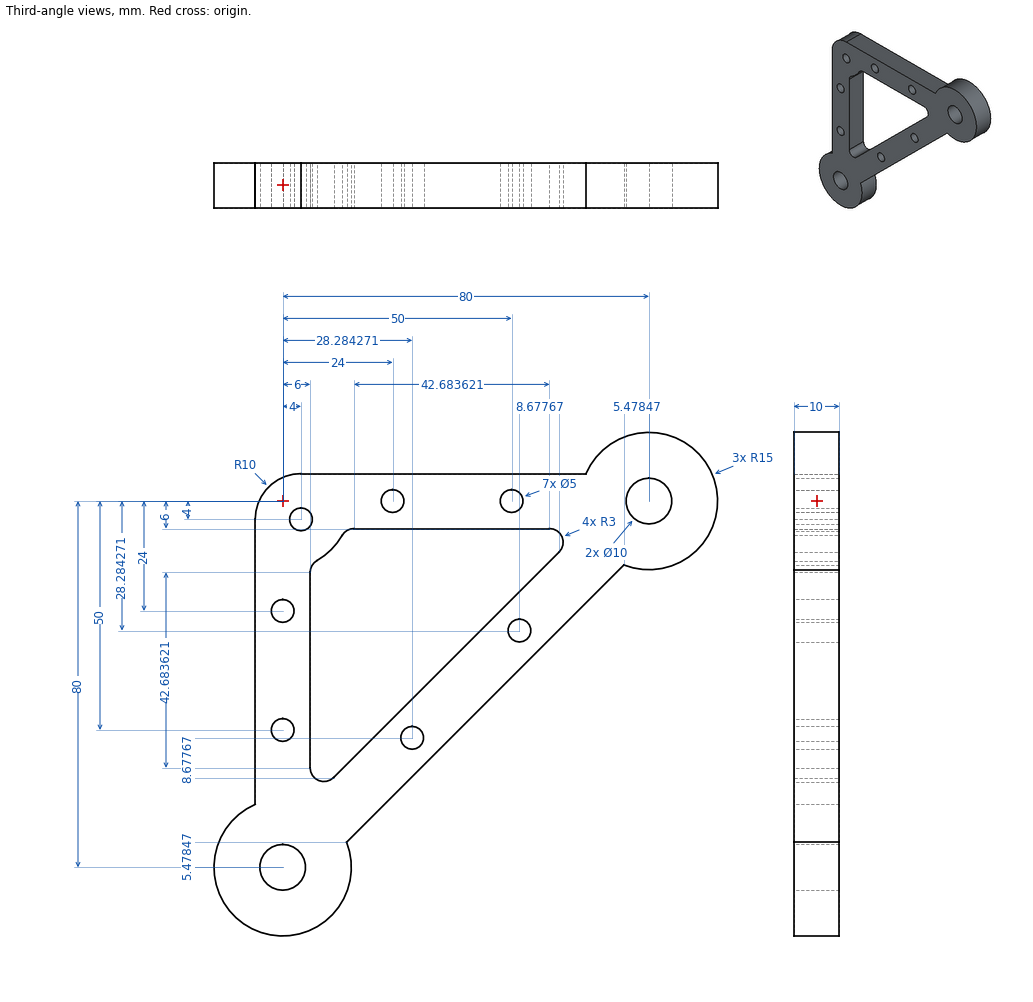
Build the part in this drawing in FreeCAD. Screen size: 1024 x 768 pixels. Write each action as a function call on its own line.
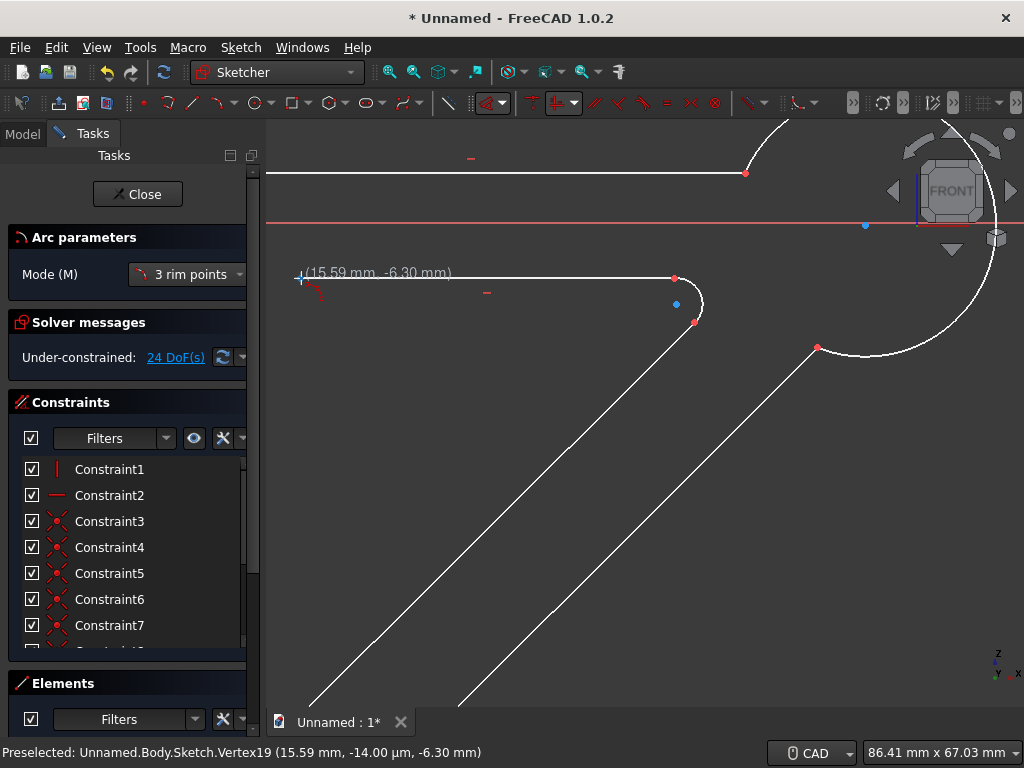
scroll(599, 254, down, 4)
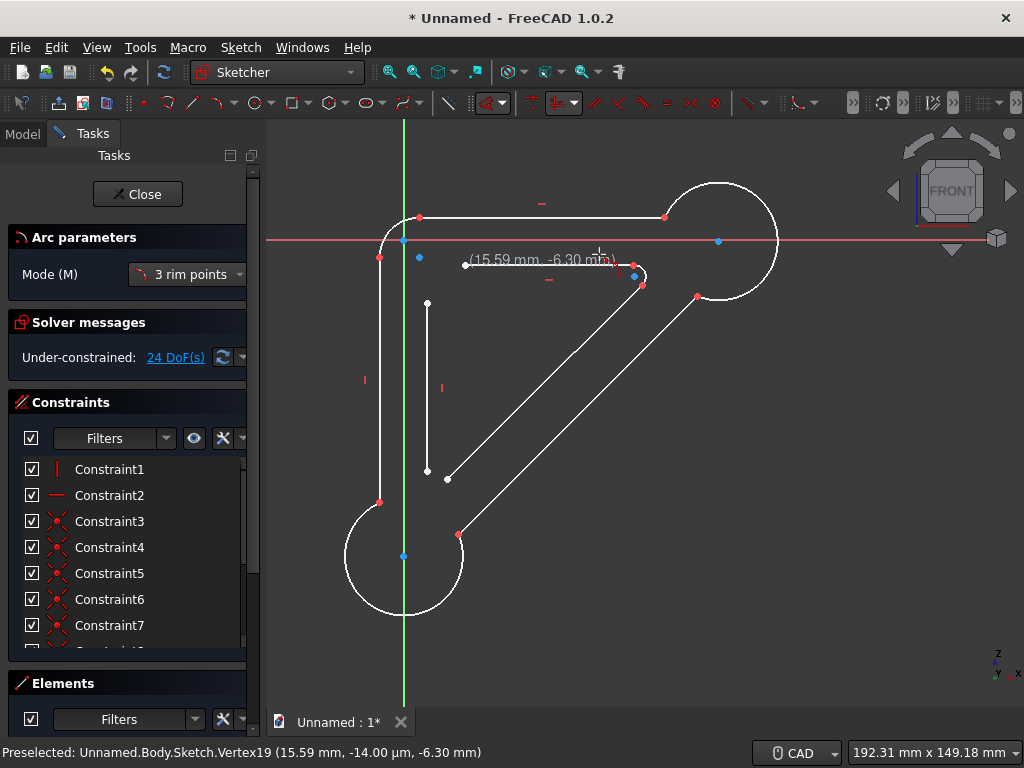
scroll(455, 270, up, 2)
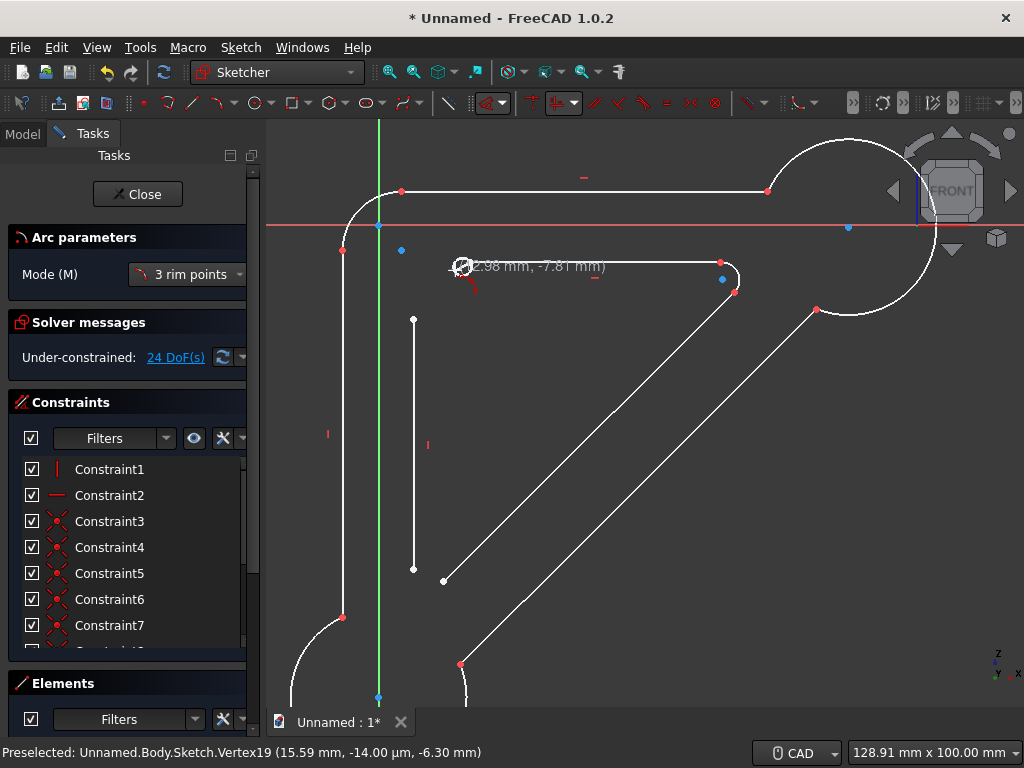
click(455, 270)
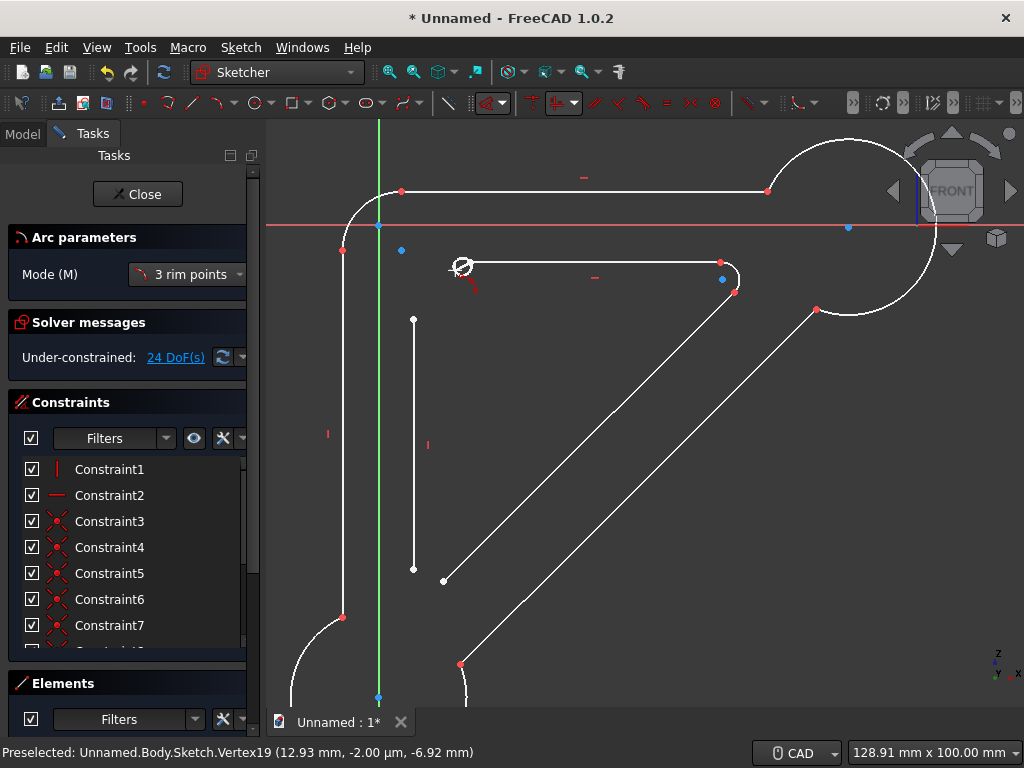
scroll(461, 263, up, 10)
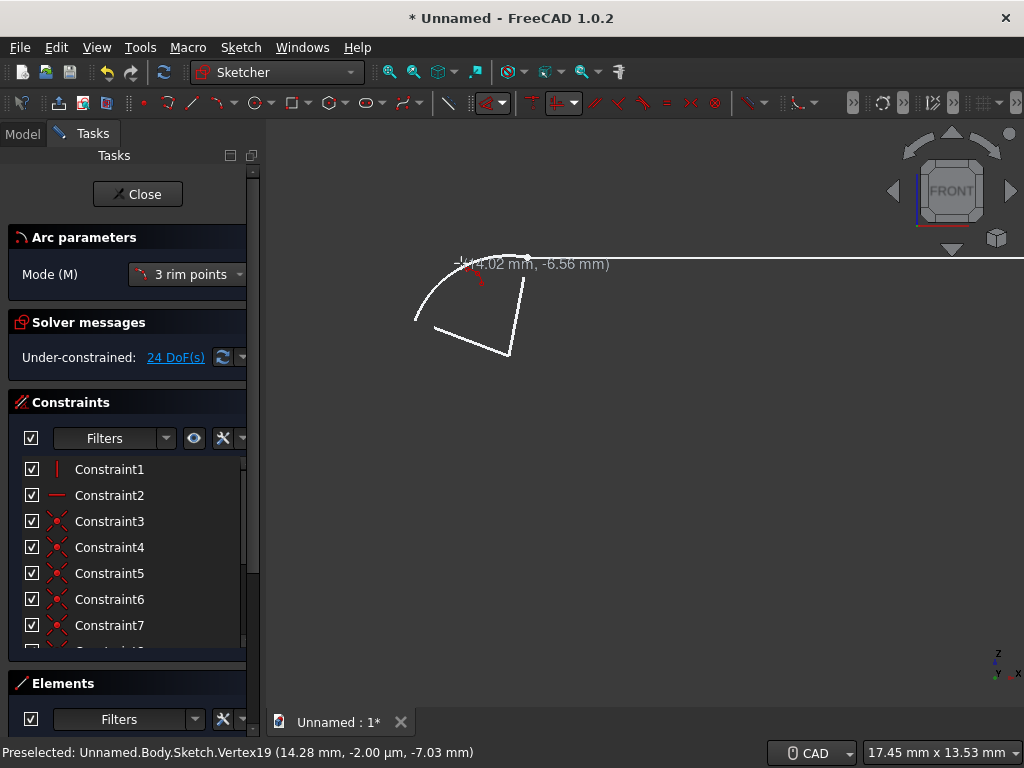
click(462, 262)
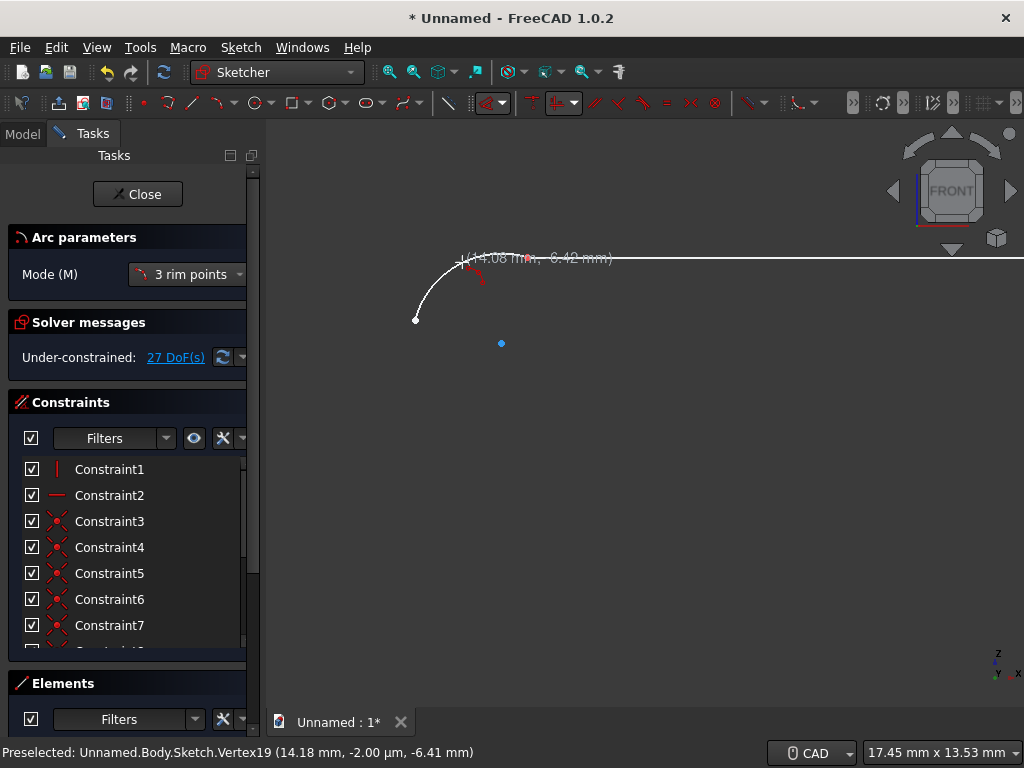
scroll(459, 265, down, 12)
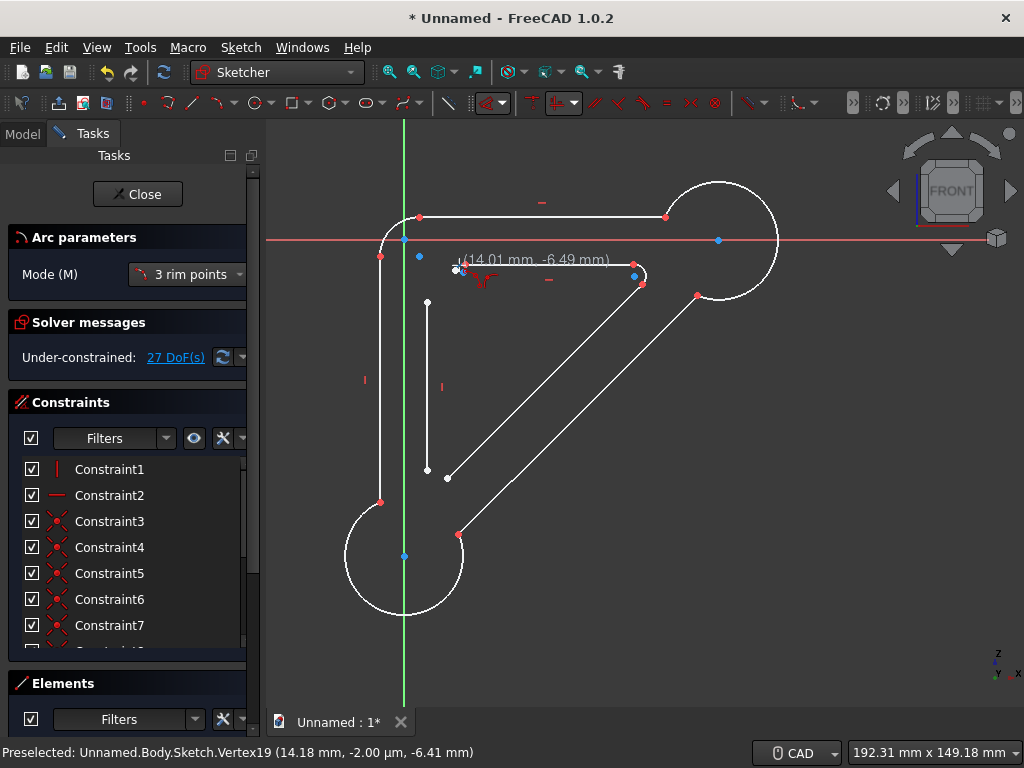
scroll(455, 269, up, 2)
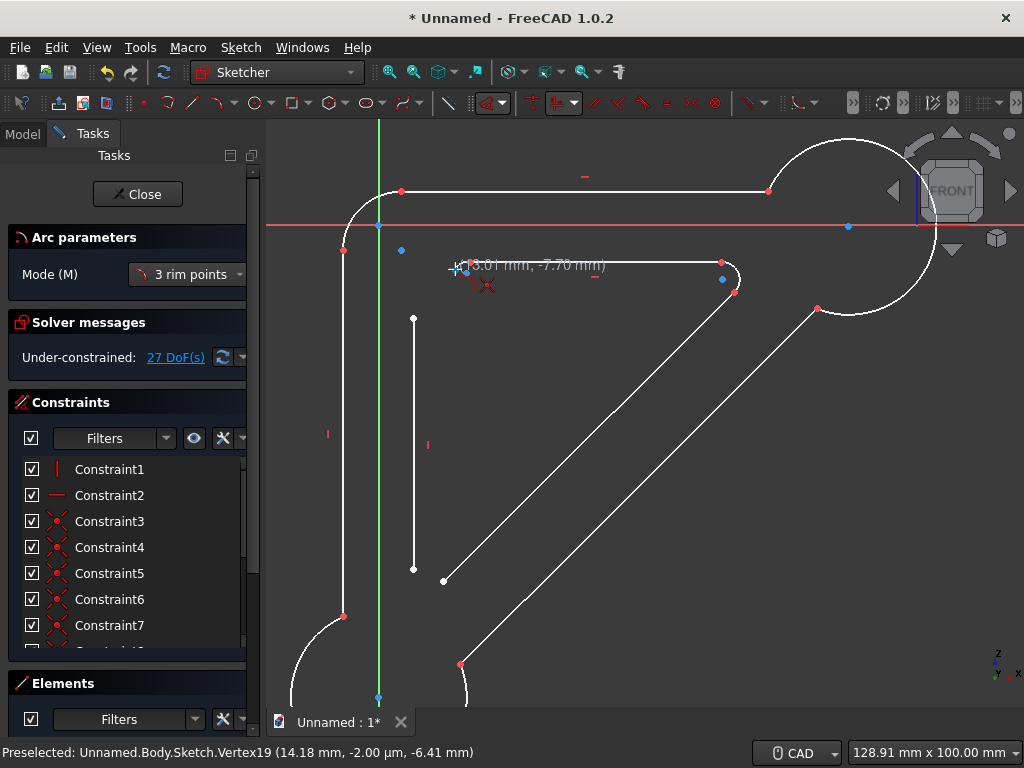
click(455, 271)
click(423, 302)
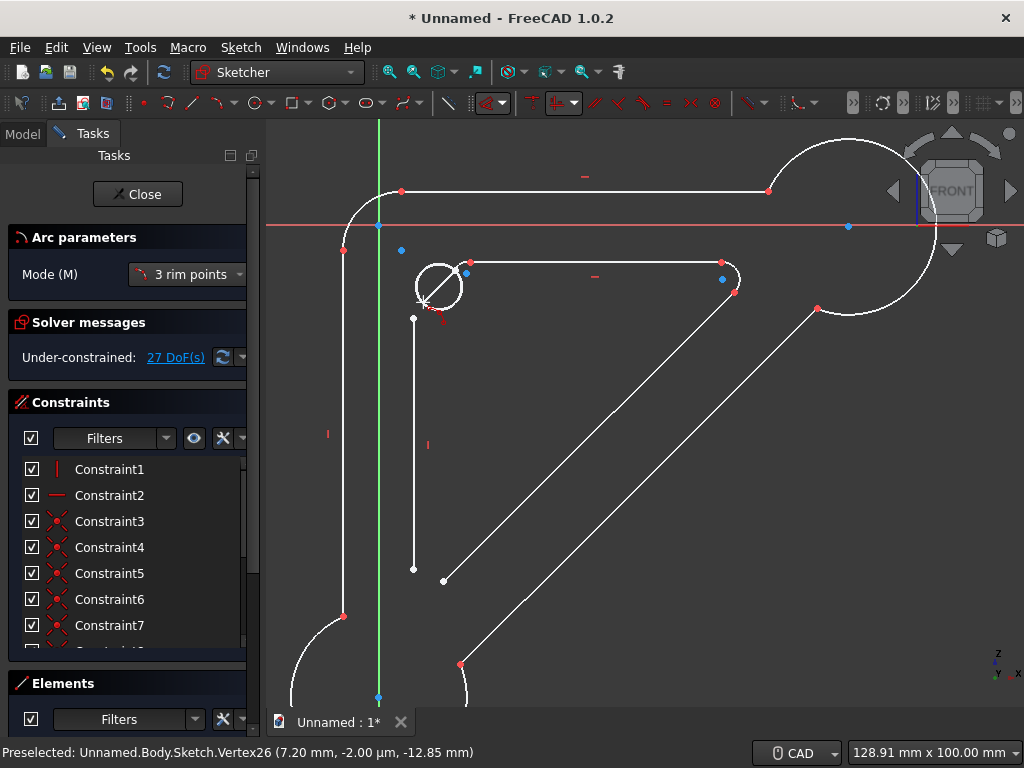
scroll(441, 288, up, 9)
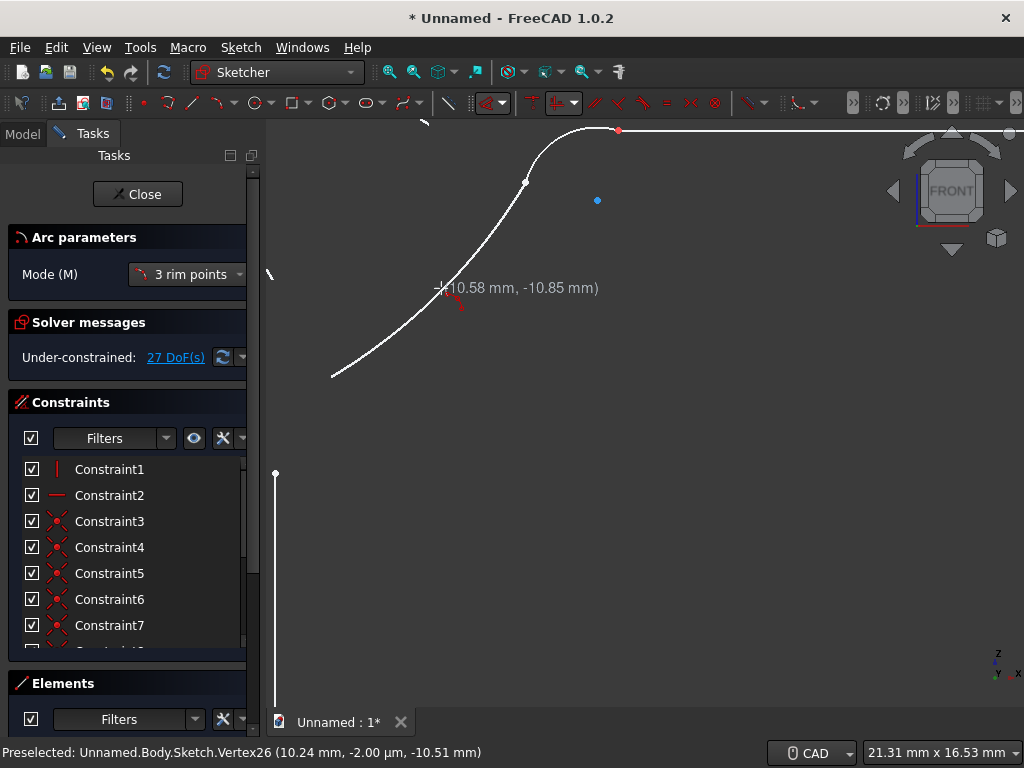
click(441, 284)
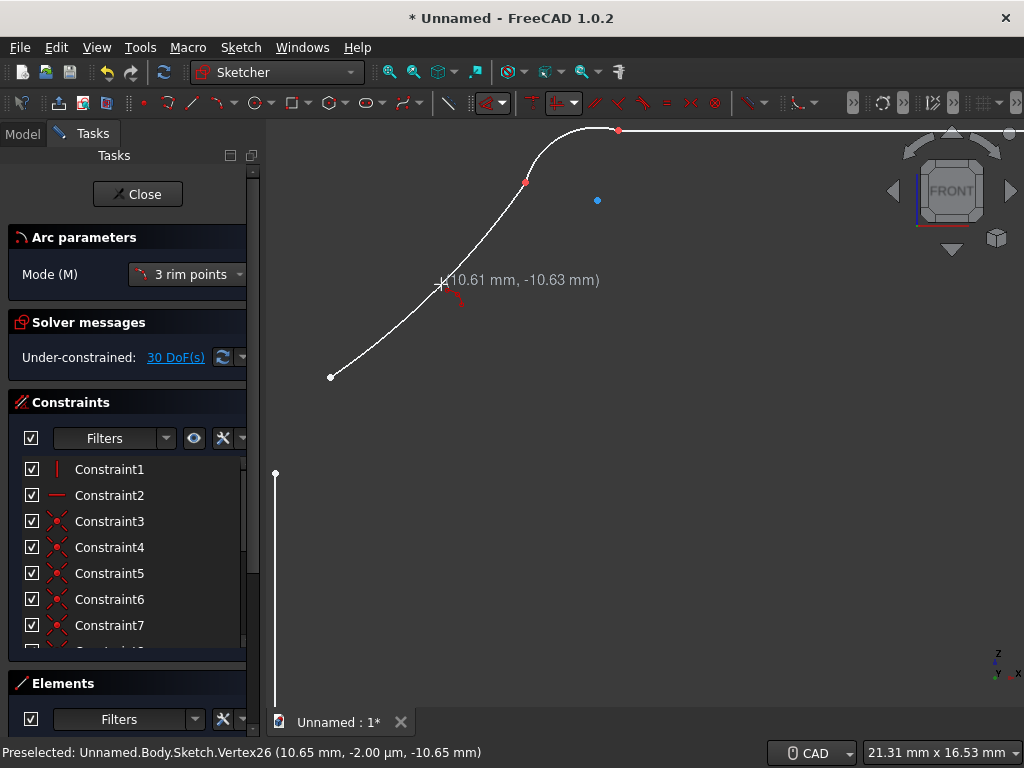
scroll(446, 281, down, 11)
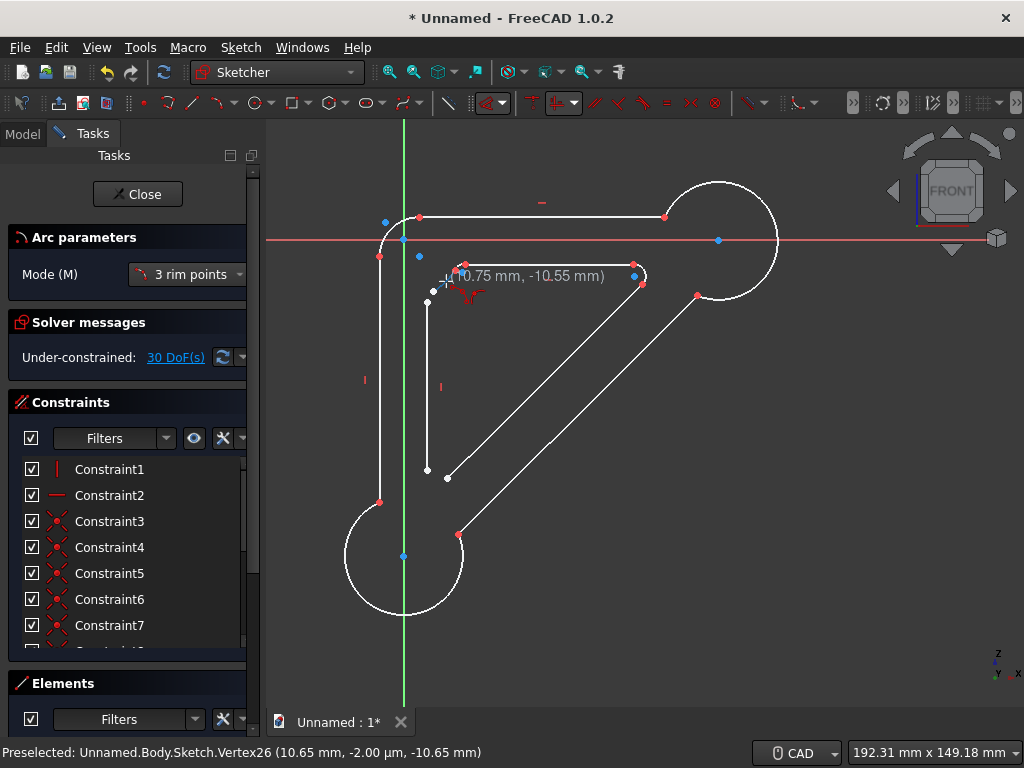
scroll(433, 291, up, 2)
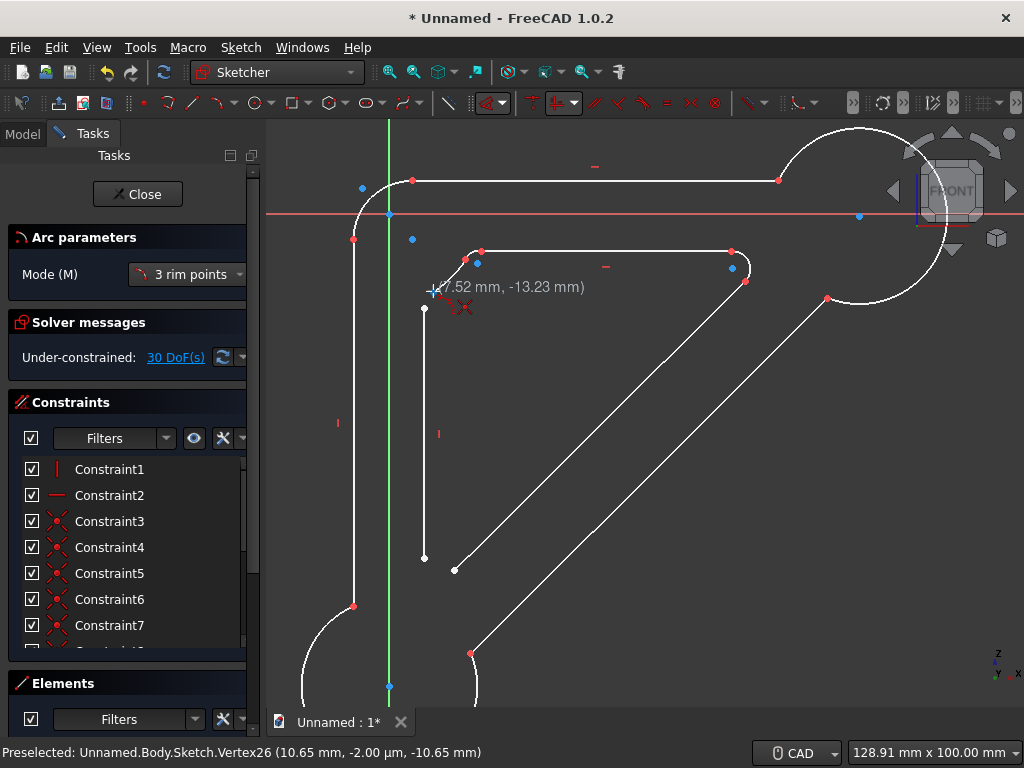
click(434, 292)
click(424, 308)